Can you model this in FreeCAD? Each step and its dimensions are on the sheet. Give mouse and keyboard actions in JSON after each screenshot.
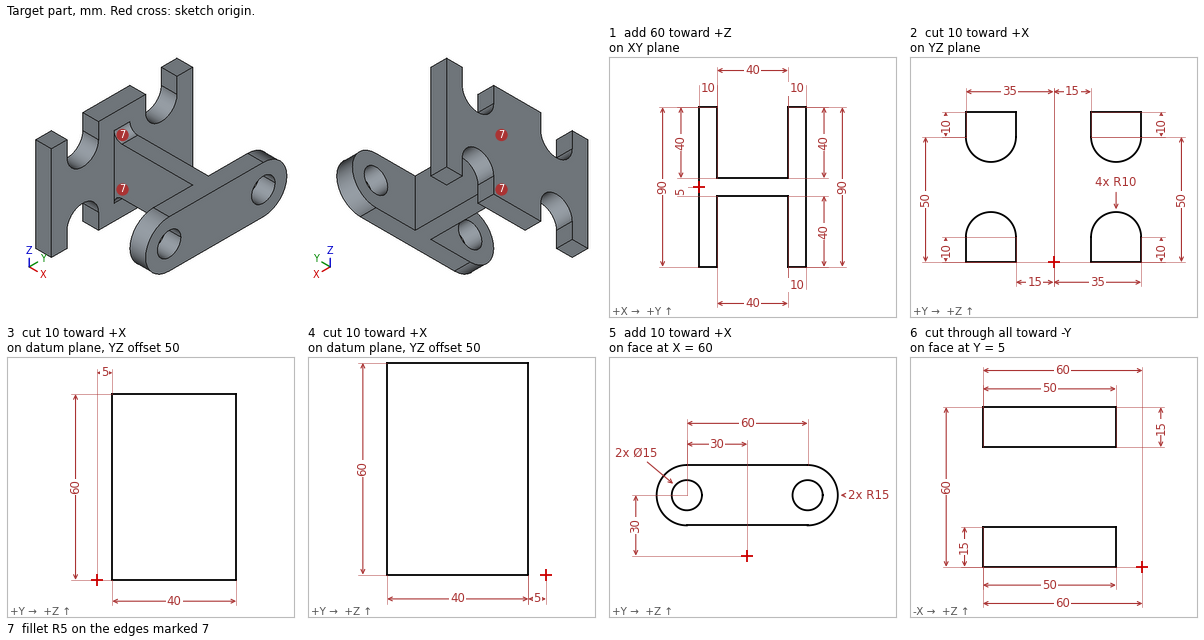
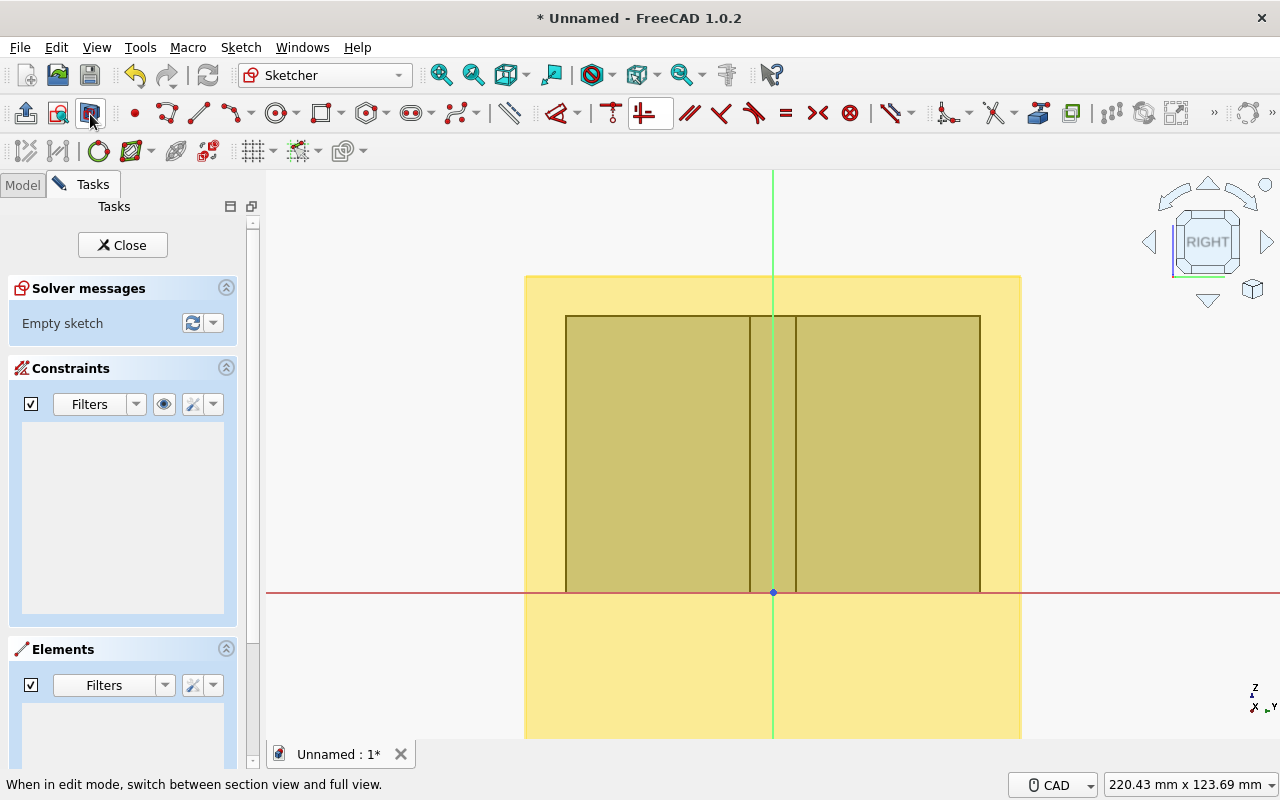
{"action": "left_click", "coordinate": [322, 114]}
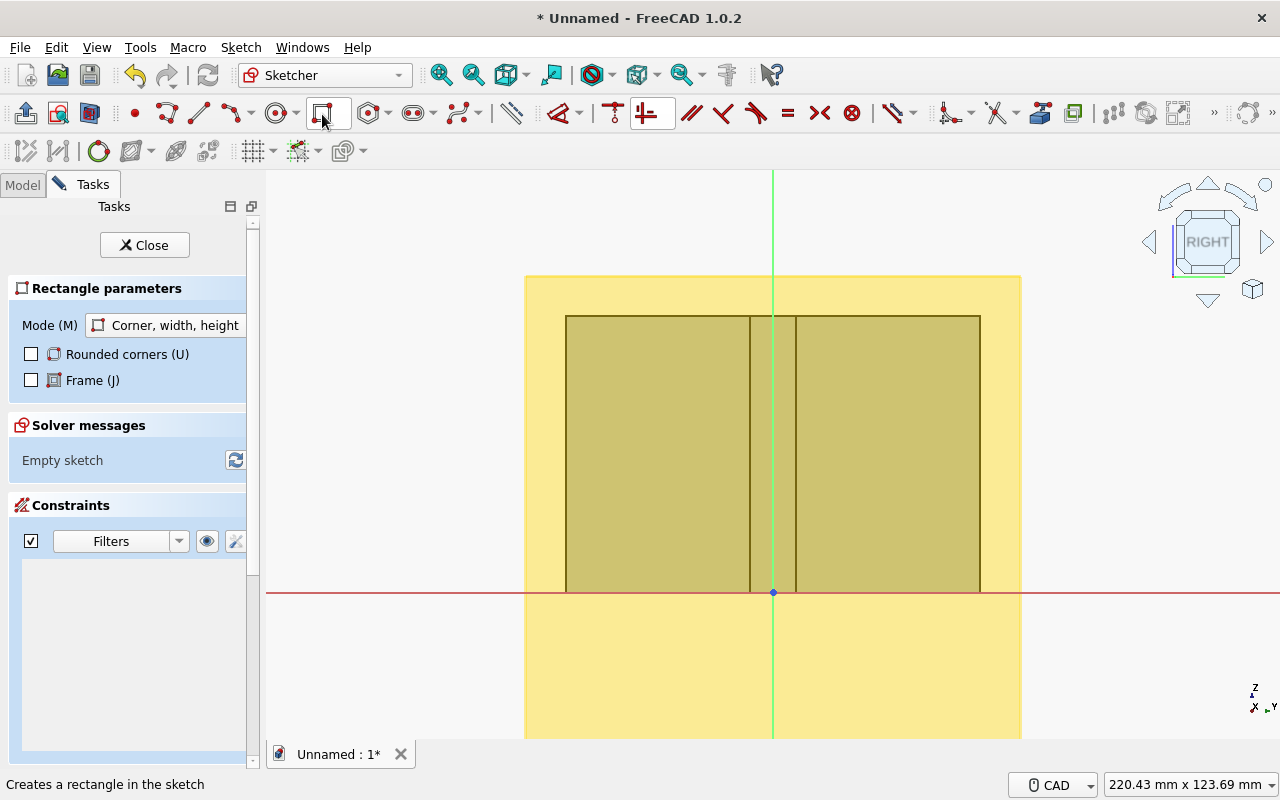
{"action": "left_click", "coordinate": [796, 316]}
{"action": "left_click", "coordinate": [980, 593]}
{"action": "key", "text": "Escape"}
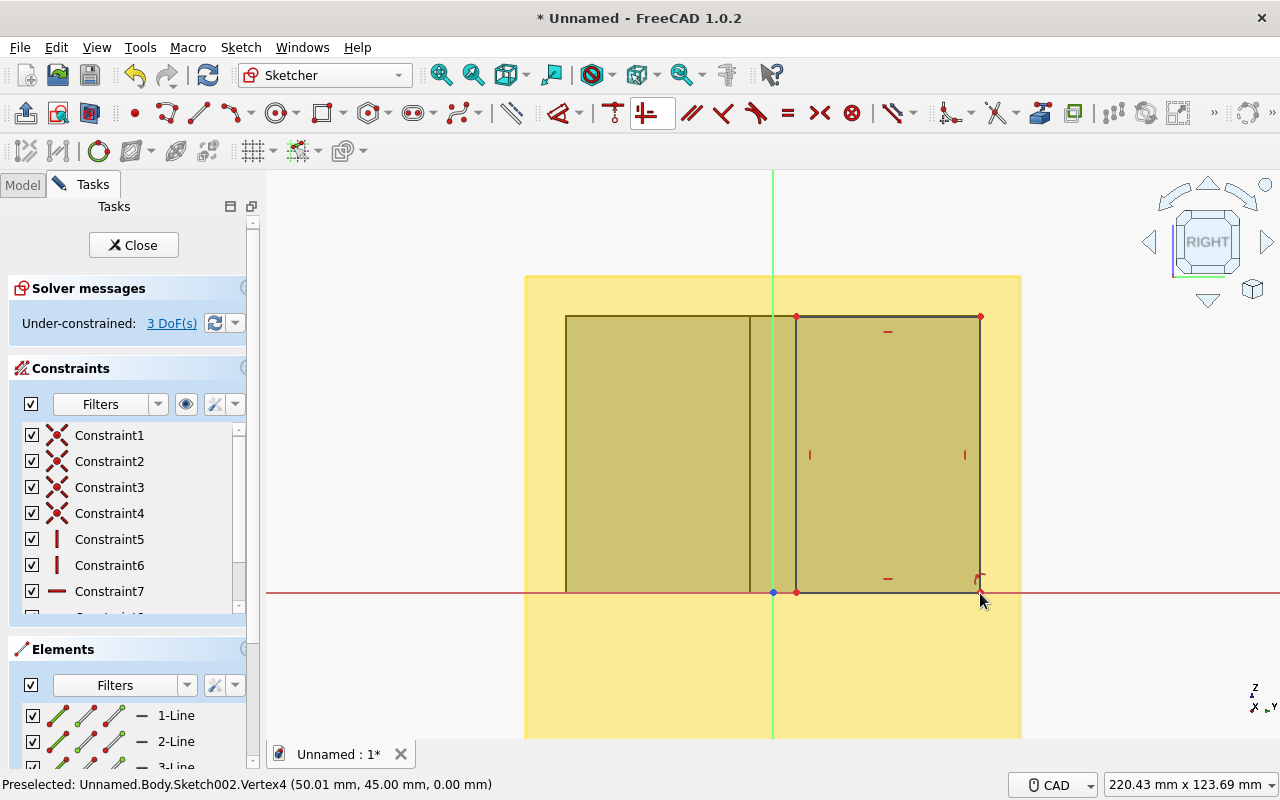
{"action": "left_click", "coordinate": [558, 114]}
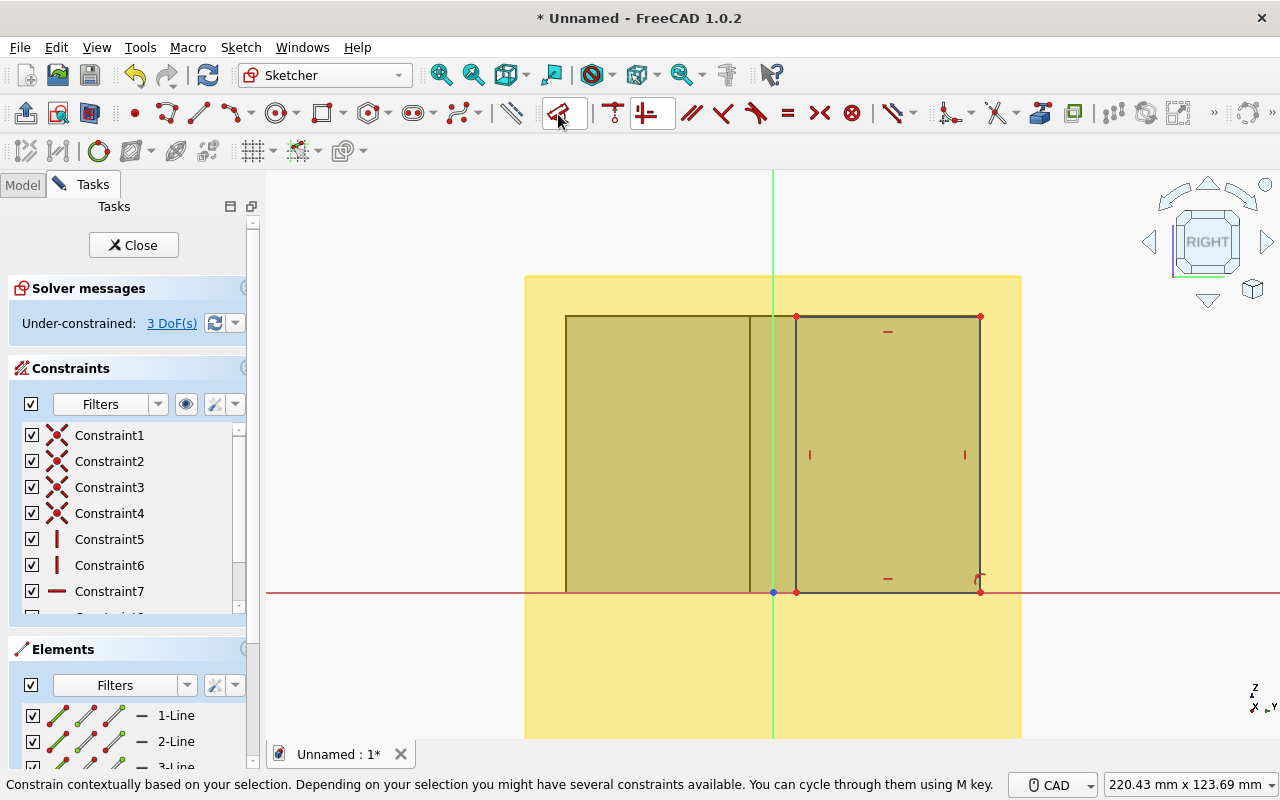
{"action": "left_click", "coordinate": [796, 400]}
{"action": "left_click", "coordinate": [830, 455]}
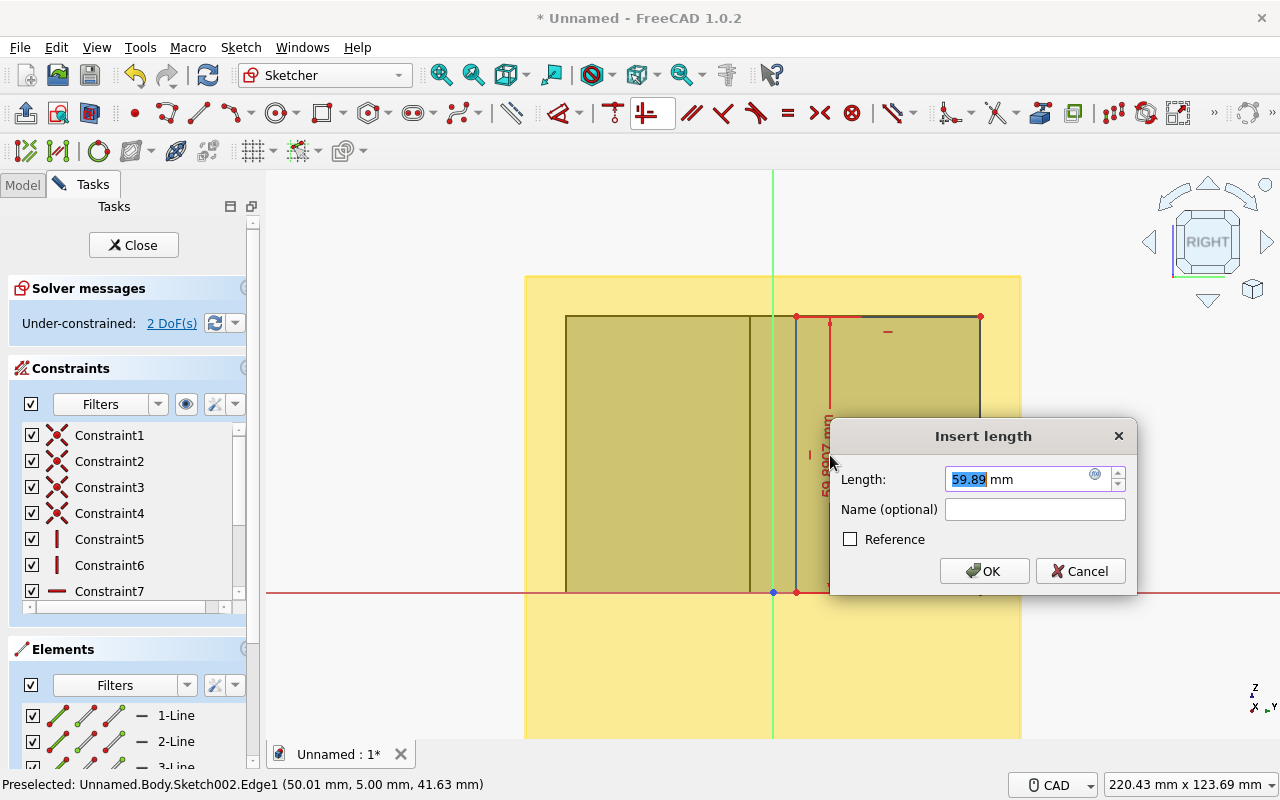
{"action": "type", "text": "60"}
{"action": "key", "text": "Return"}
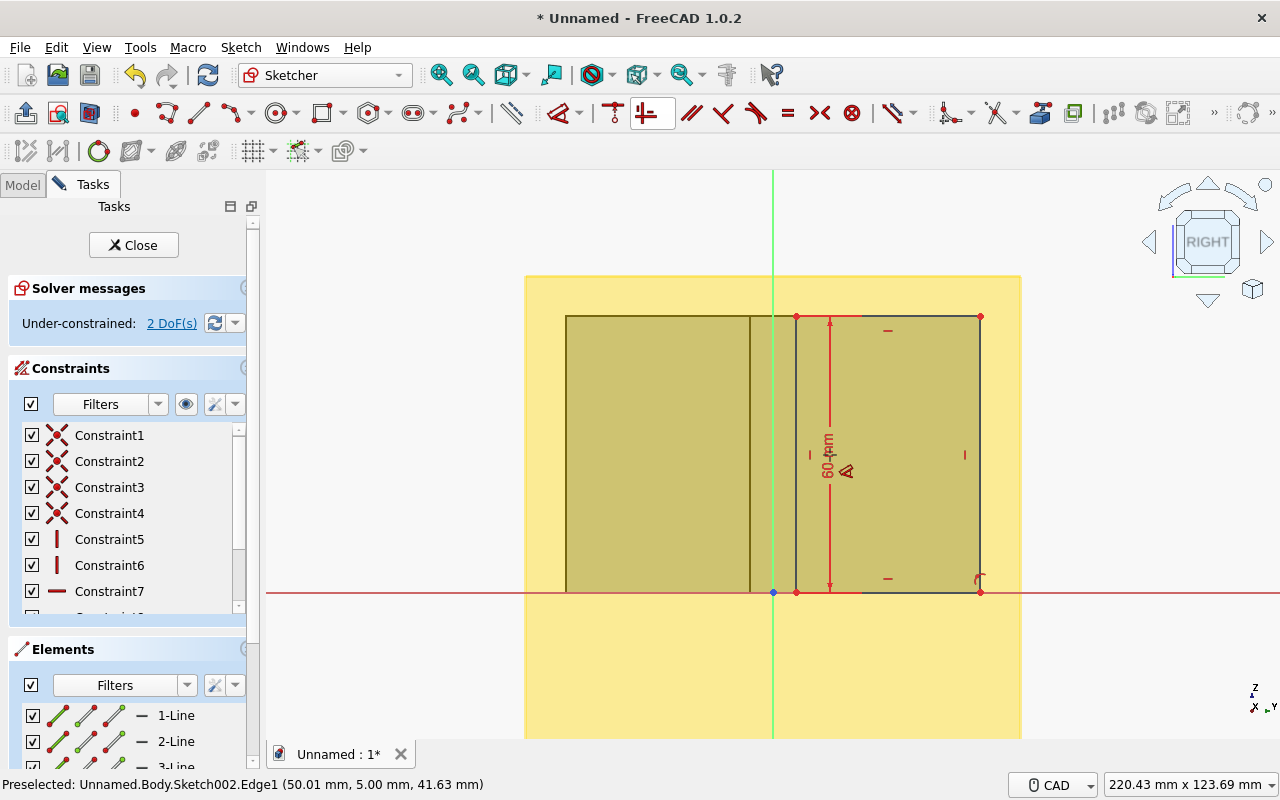
{"action": "left_click", "coordinate": [851, 593]}
{"action": "left_click", "coordinate": [888, 627]}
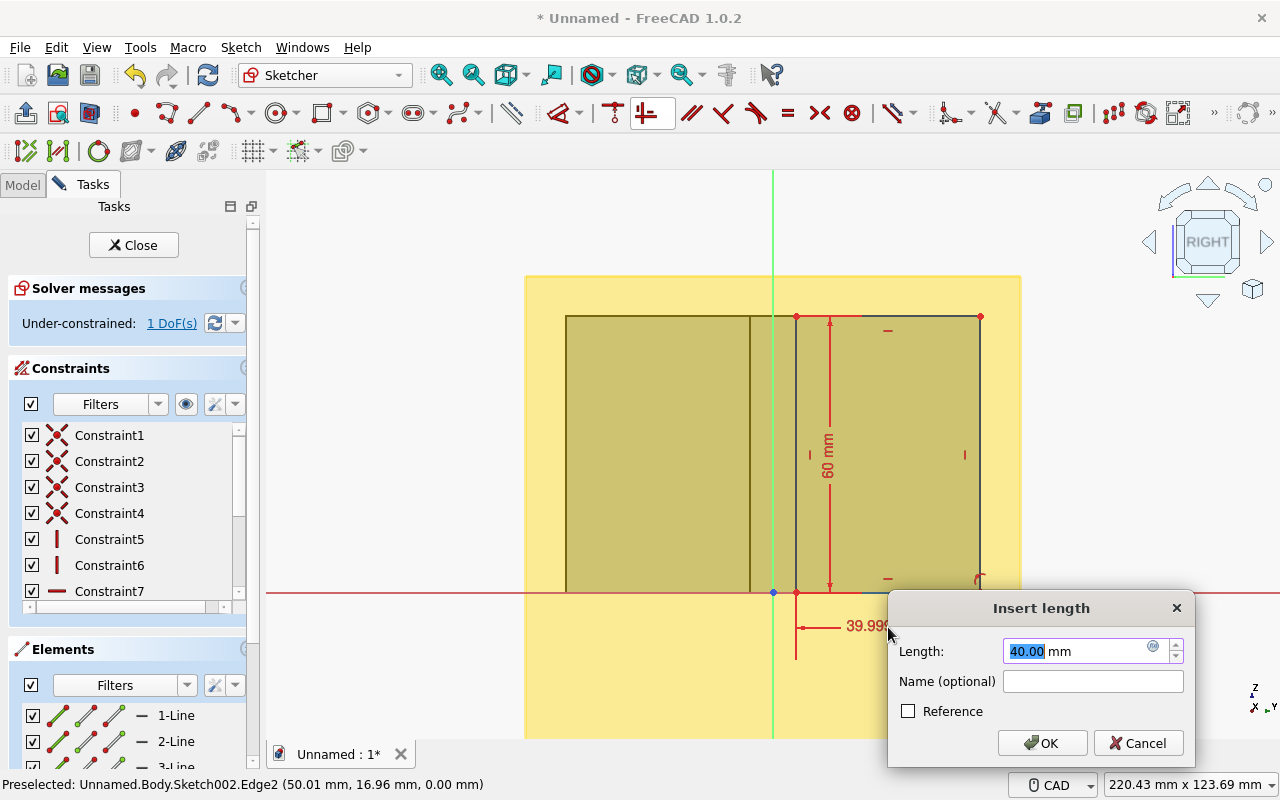
{"action": "type", "text": "40"}
{"action": "key", "text": "Return"}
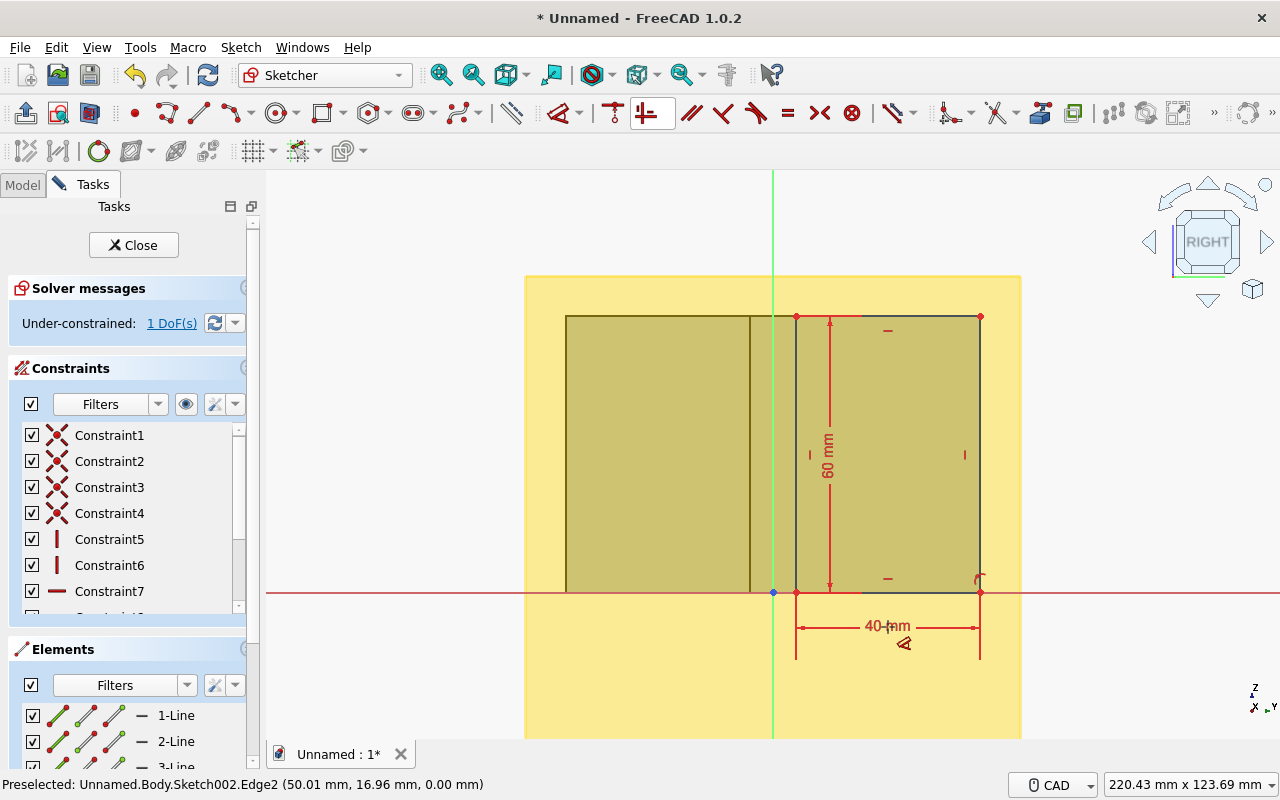
{"action": "scroll", "coordinate": [796, 316], "scroll_direction": "up", "scroll_amount": 3}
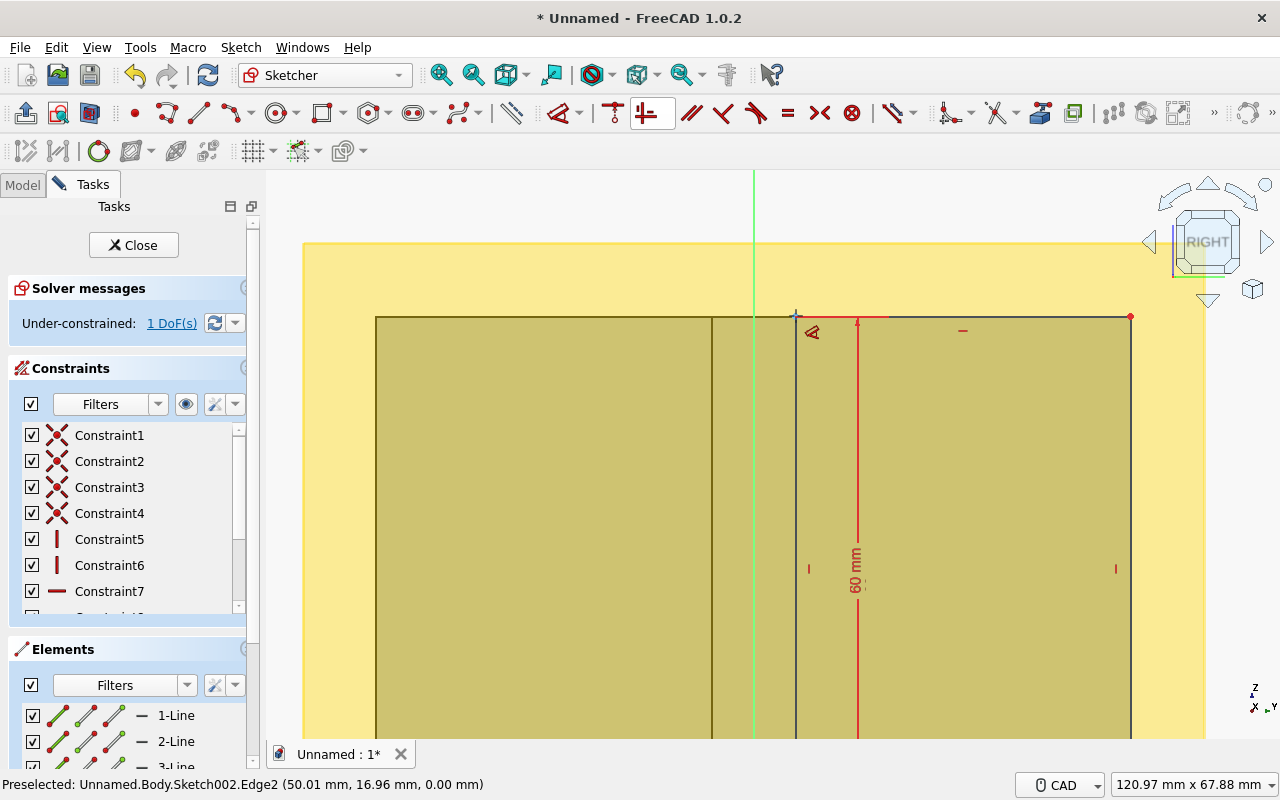
{"action": "left_click", "coordinate": [796, 317]}
{"action": "left_click", "coordinate": [775, 283]}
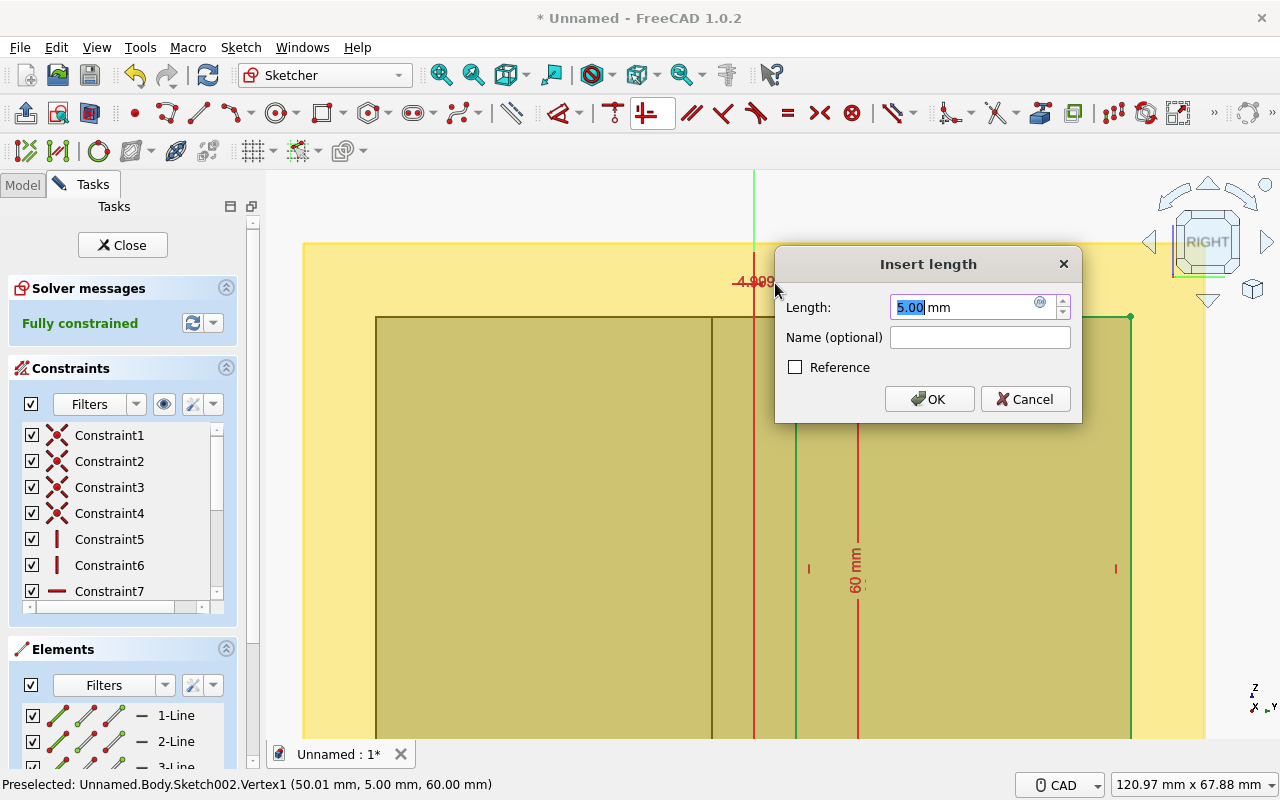
{"action": "type", "text": "5"}
{"action": "key", "text": "Return"}
{"action": "key", "text": "Escape"}